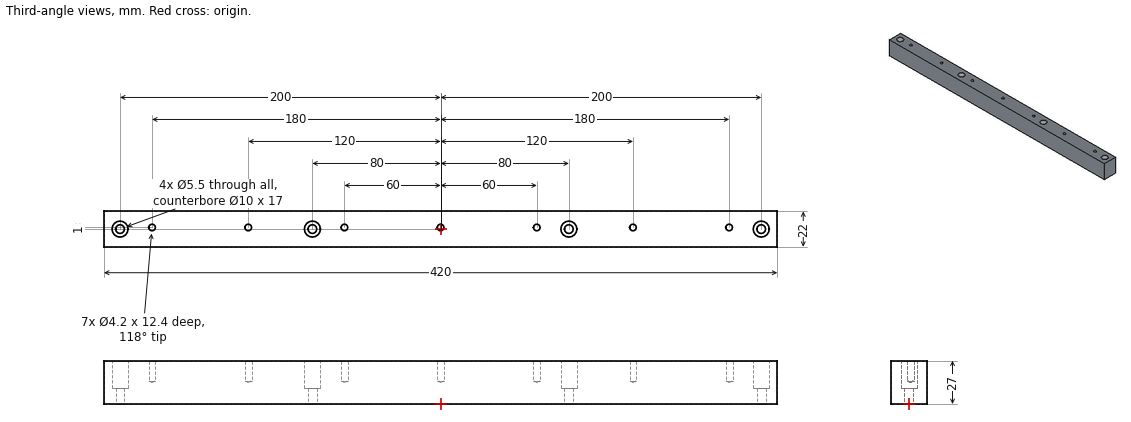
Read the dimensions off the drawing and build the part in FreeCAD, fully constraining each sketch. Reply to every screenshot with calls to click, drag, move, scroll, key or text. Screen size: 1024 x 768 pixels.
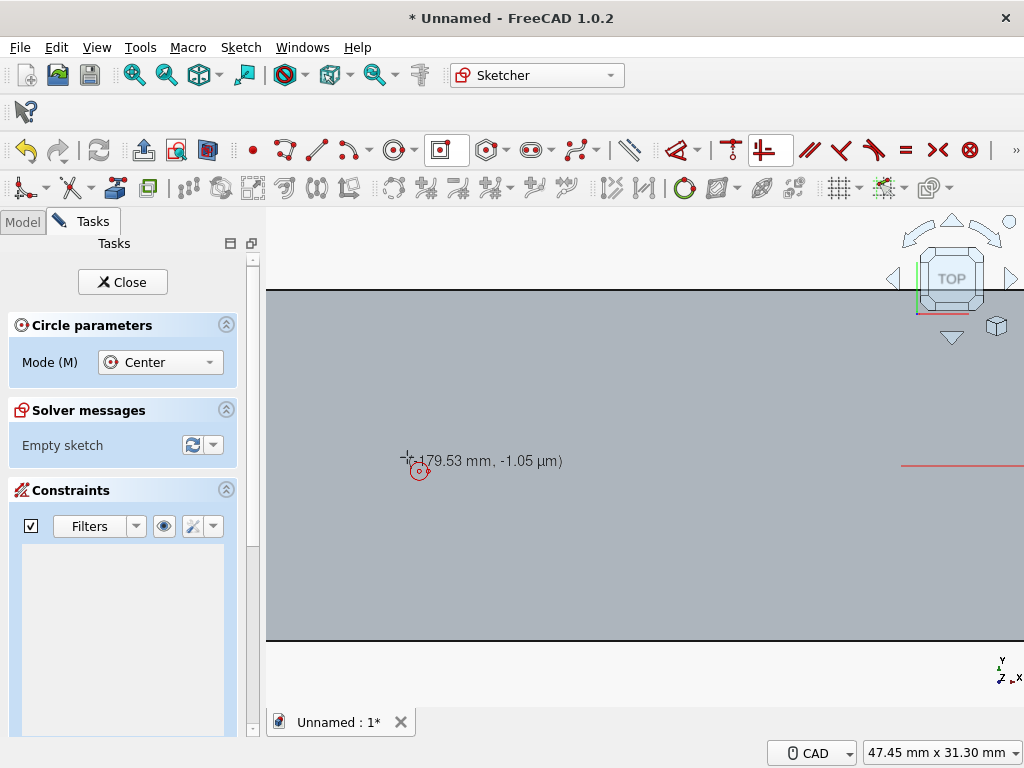
click(397, 450)
move(420, 426)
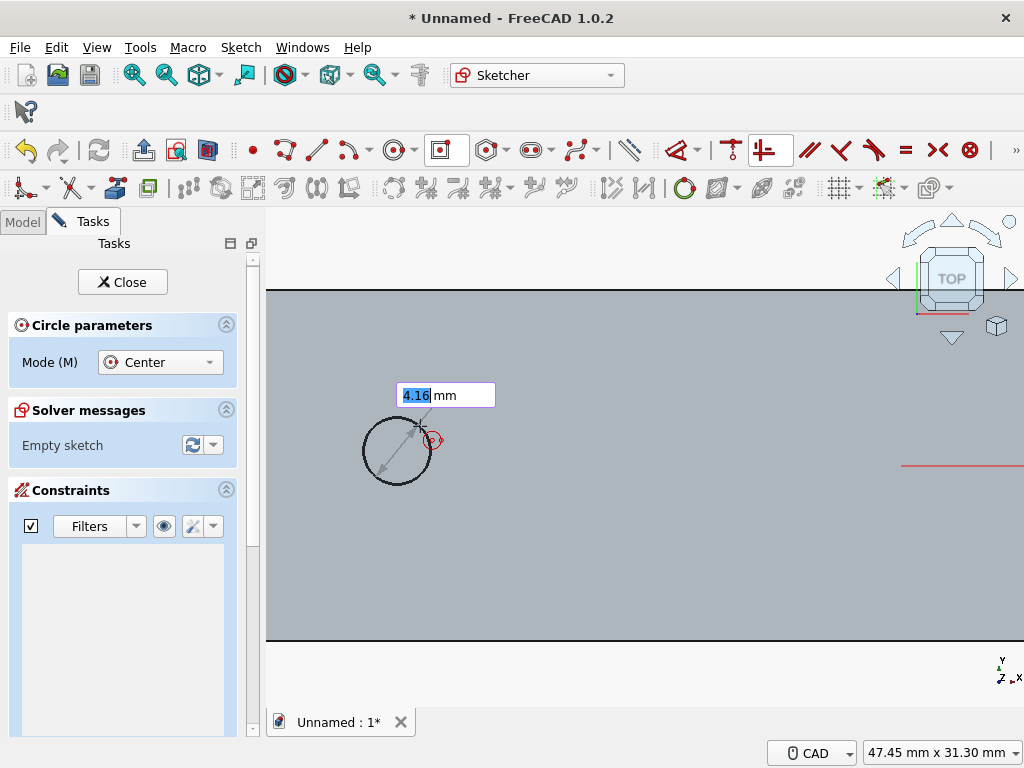
text(4.2)
key(Return)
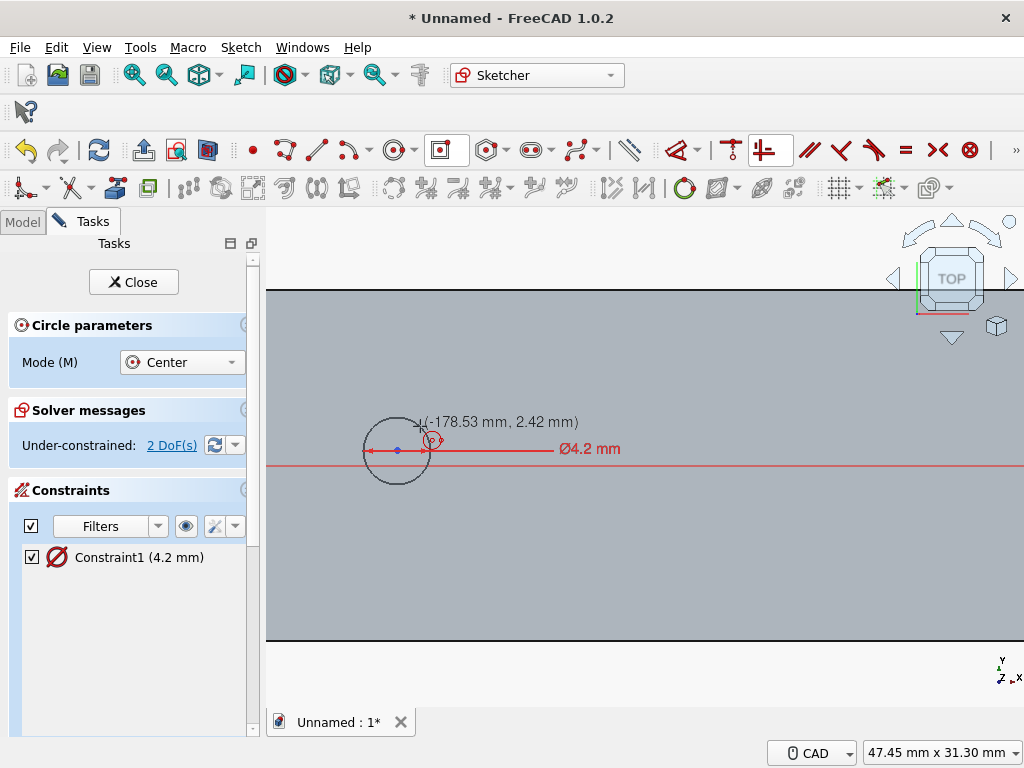
scroll(360, 458, down, 13)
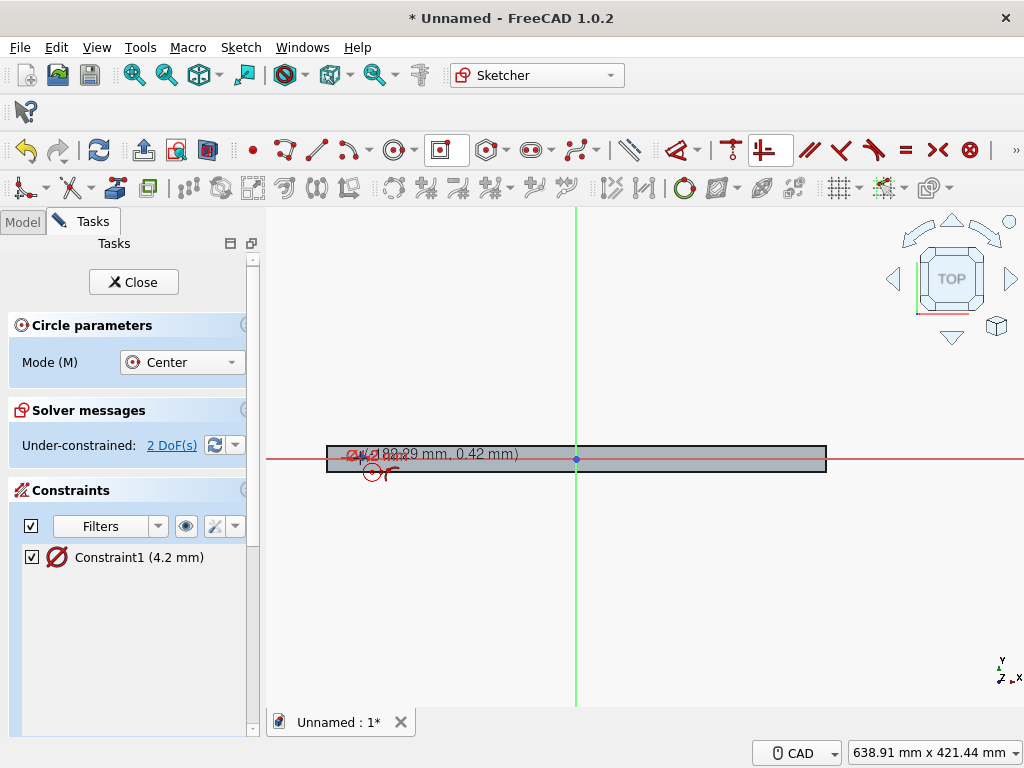
scroll(434, 458, up, 13)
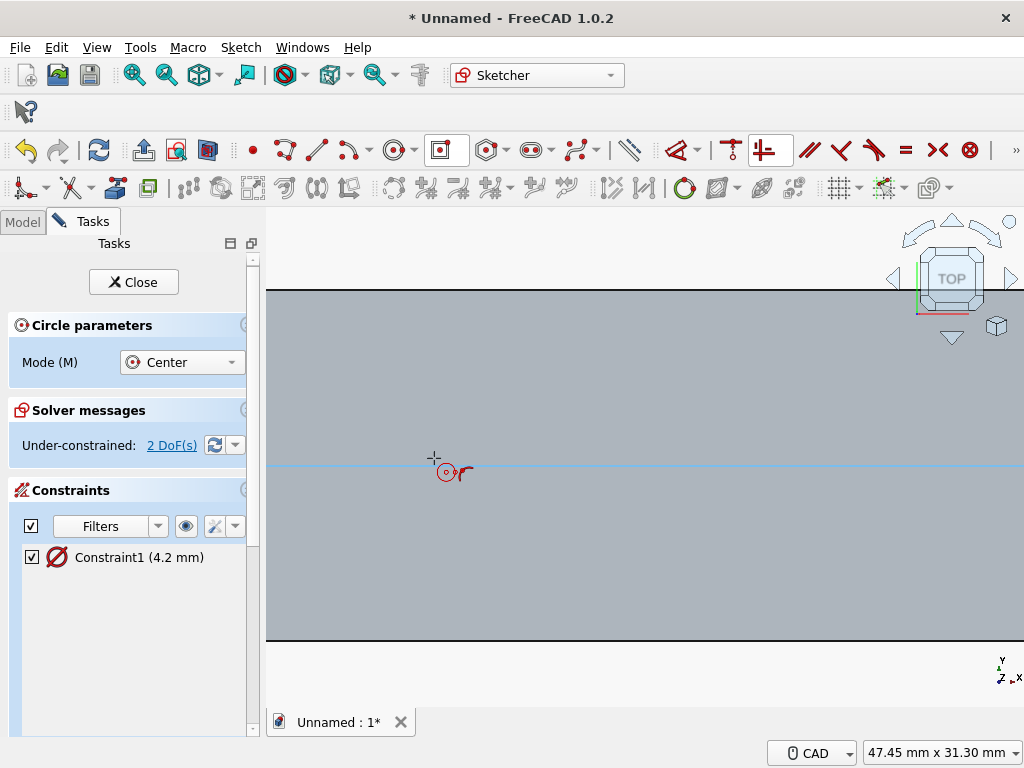
click(431, 450)
move(455, 426)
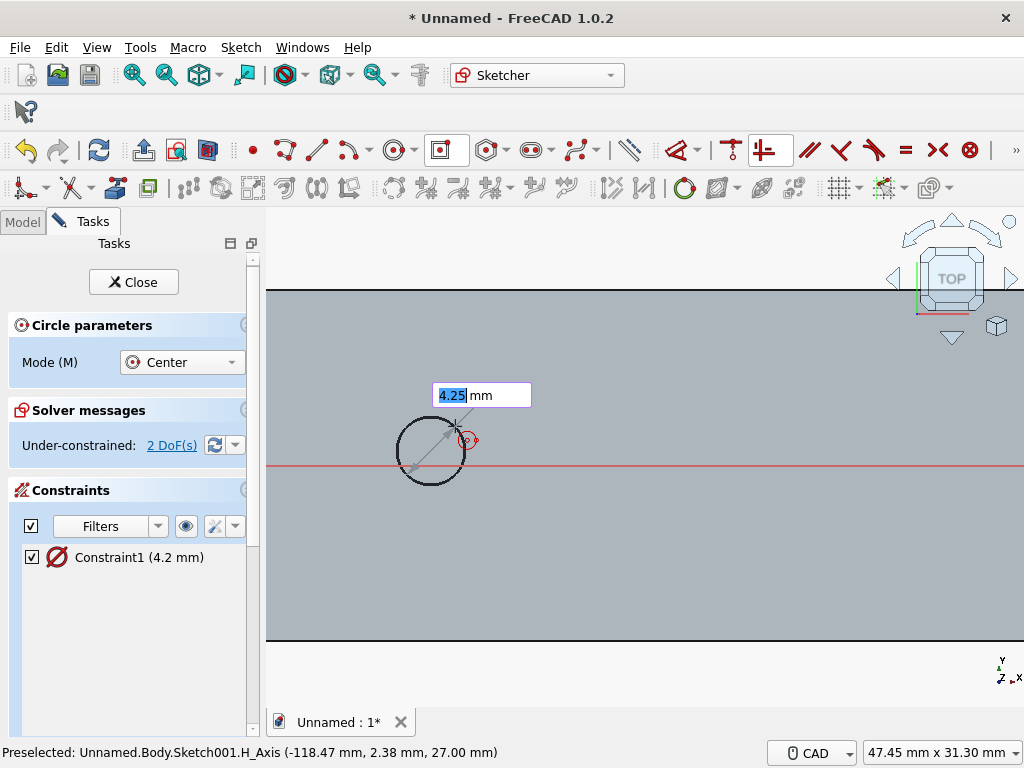
text(4.2)
key(Return)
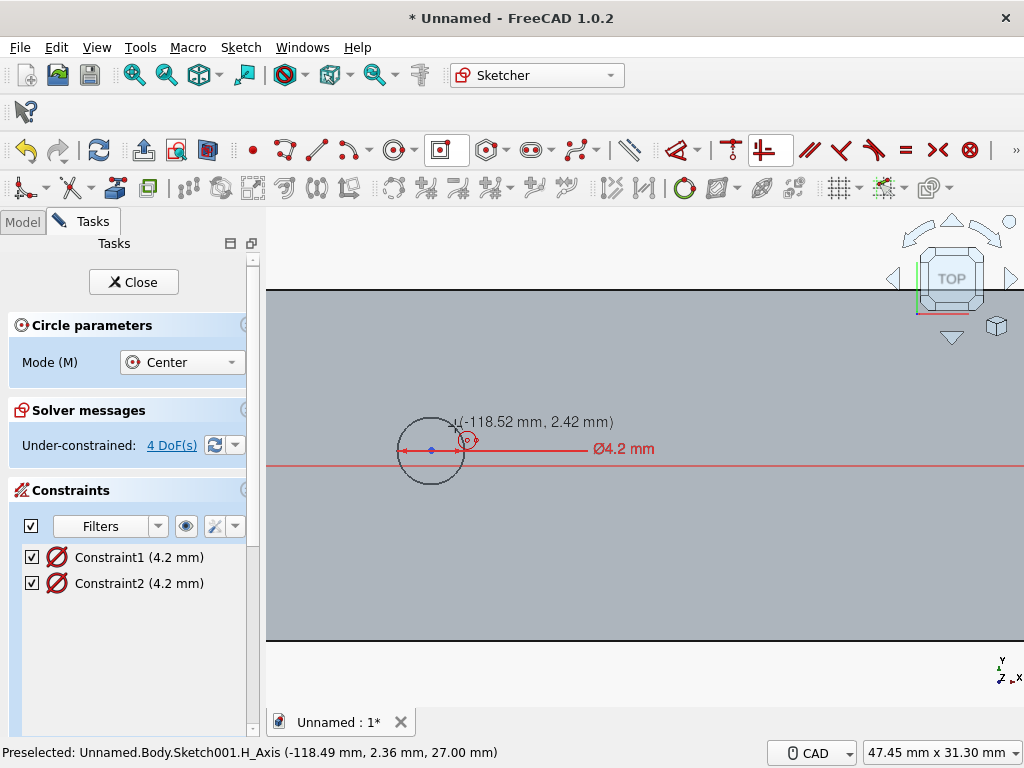
scroll(434, 458, down, 13)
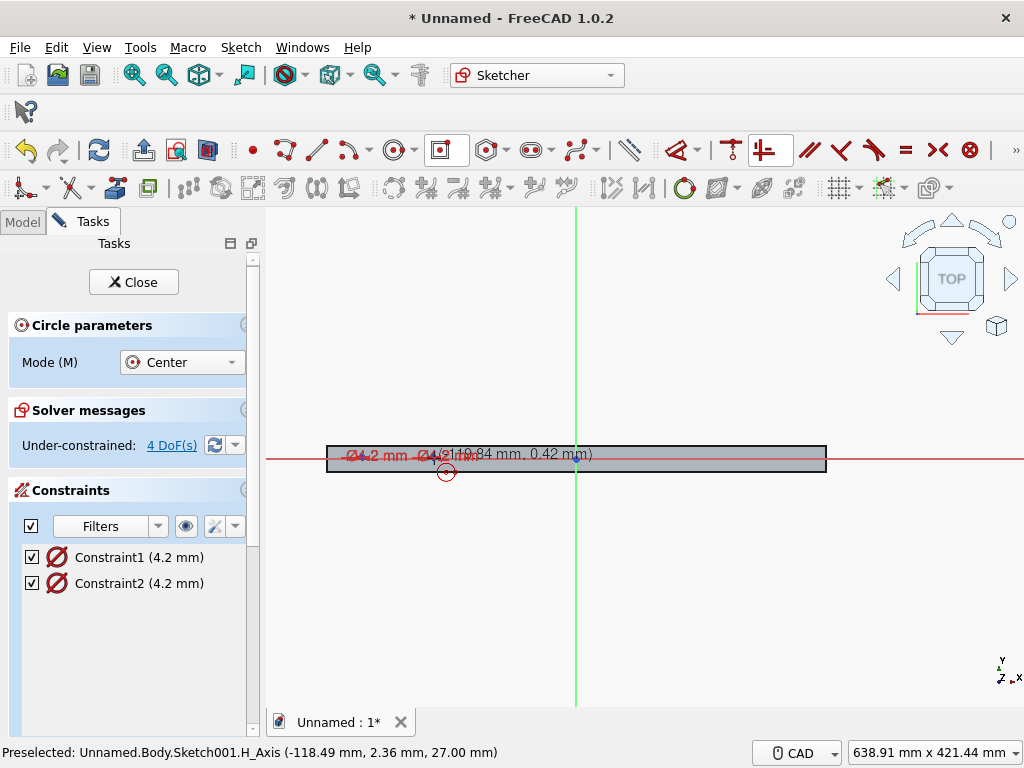
scroll(505, 458, up, 13)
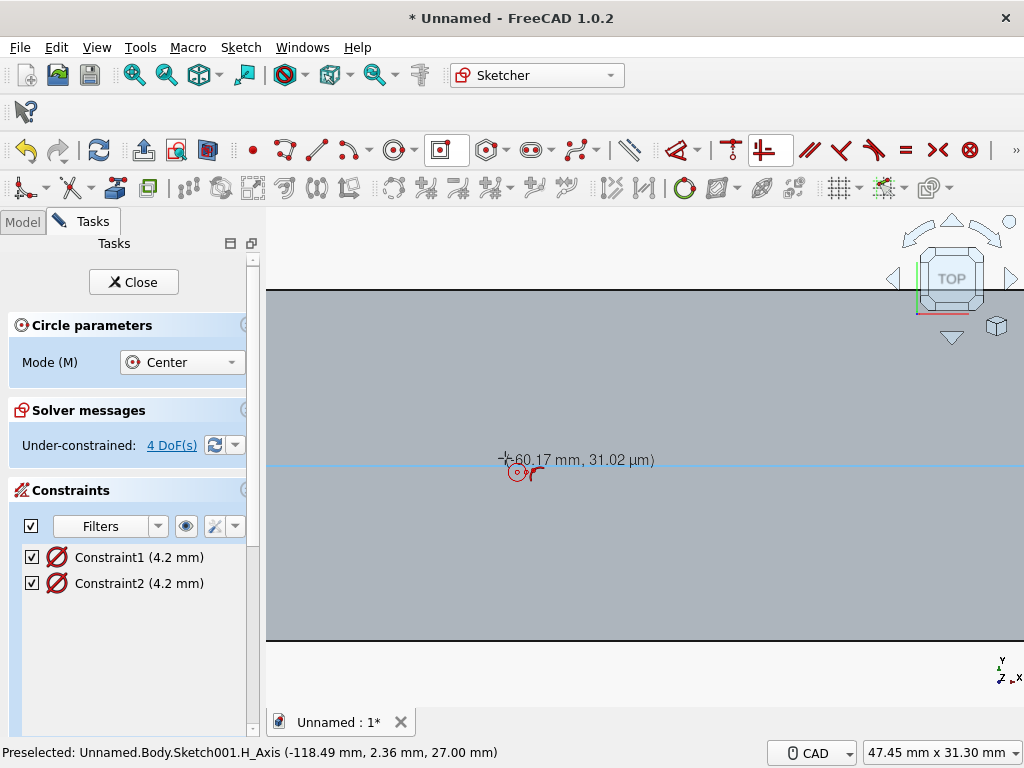
click(504, 450)
move(527, 426)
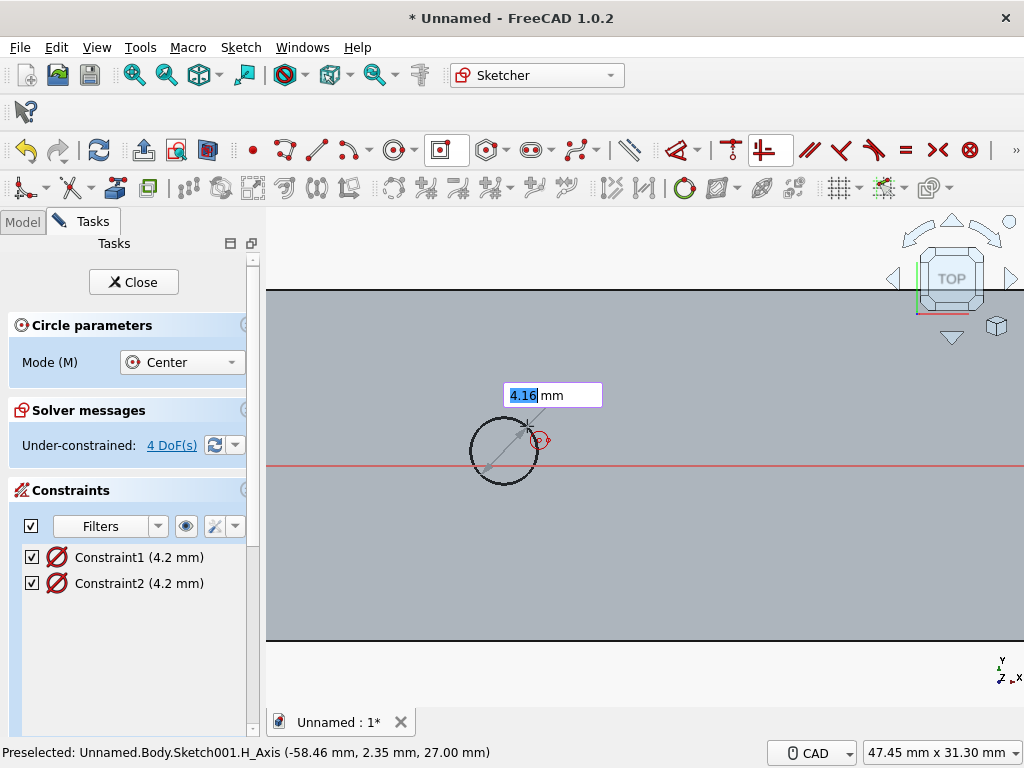
text(4.2)
key(Return)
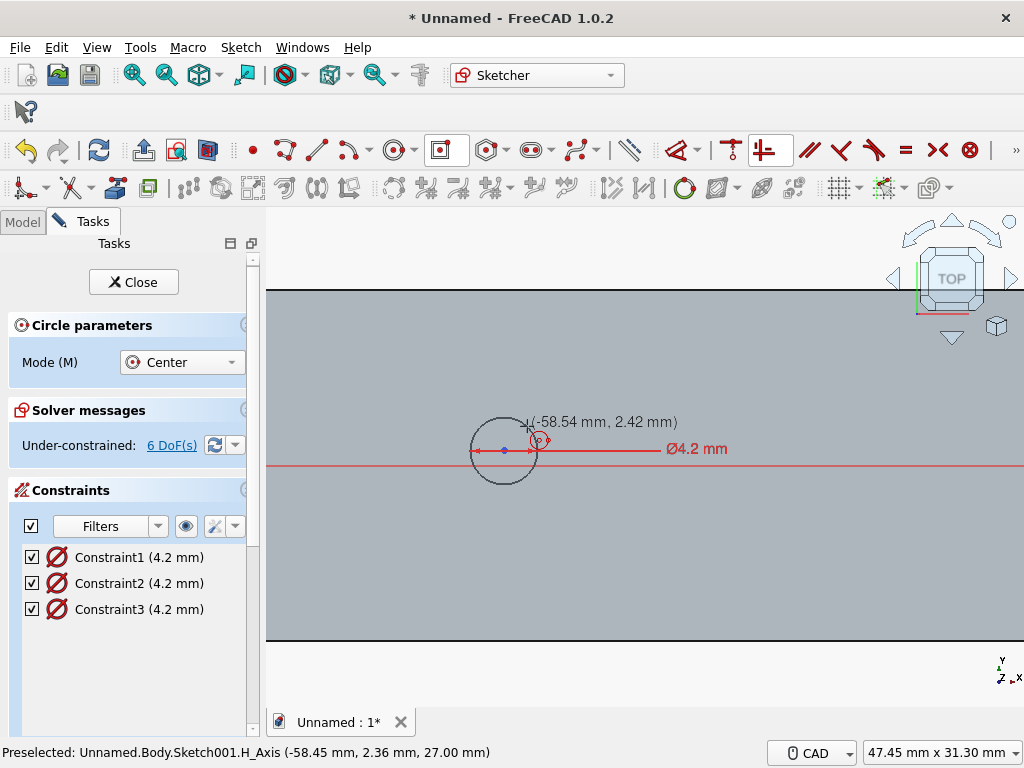
scroll(505, 458, down, 13)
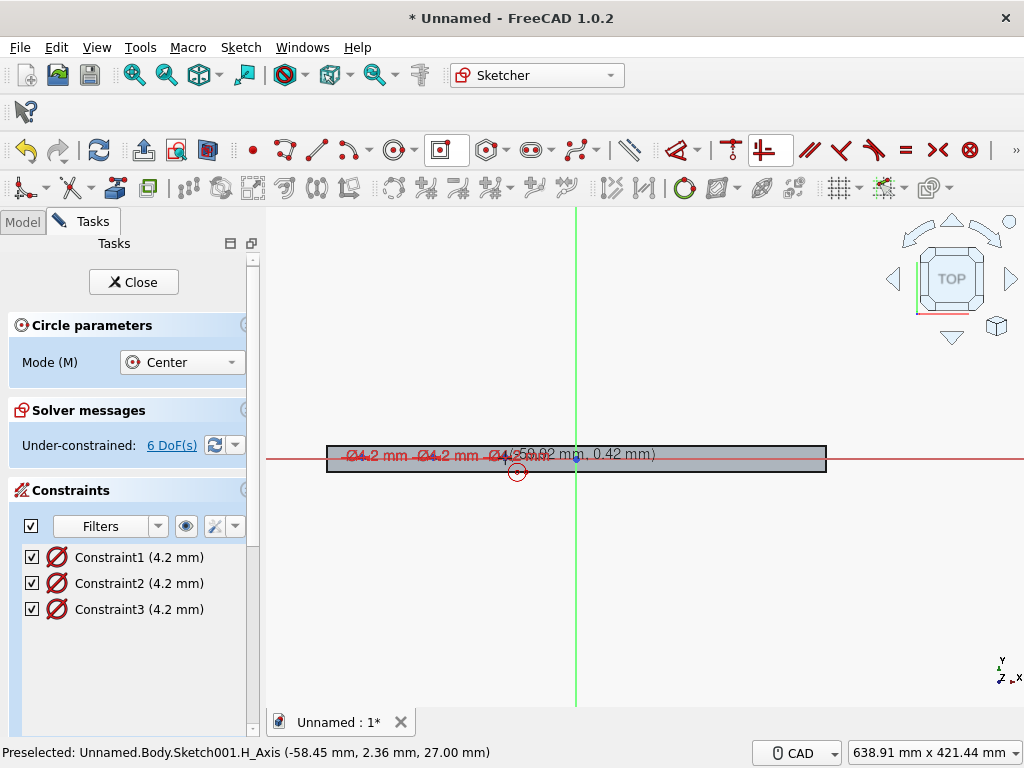
scroll(576, 458, up, 13)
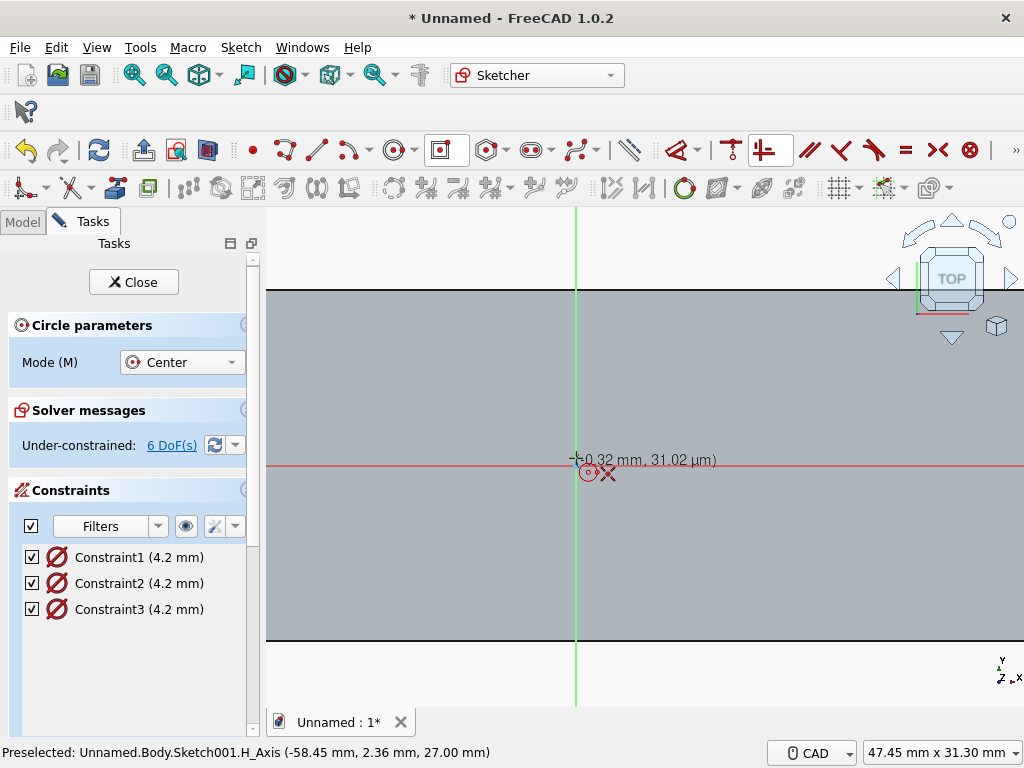
click(576, 450)
move(600, 426)